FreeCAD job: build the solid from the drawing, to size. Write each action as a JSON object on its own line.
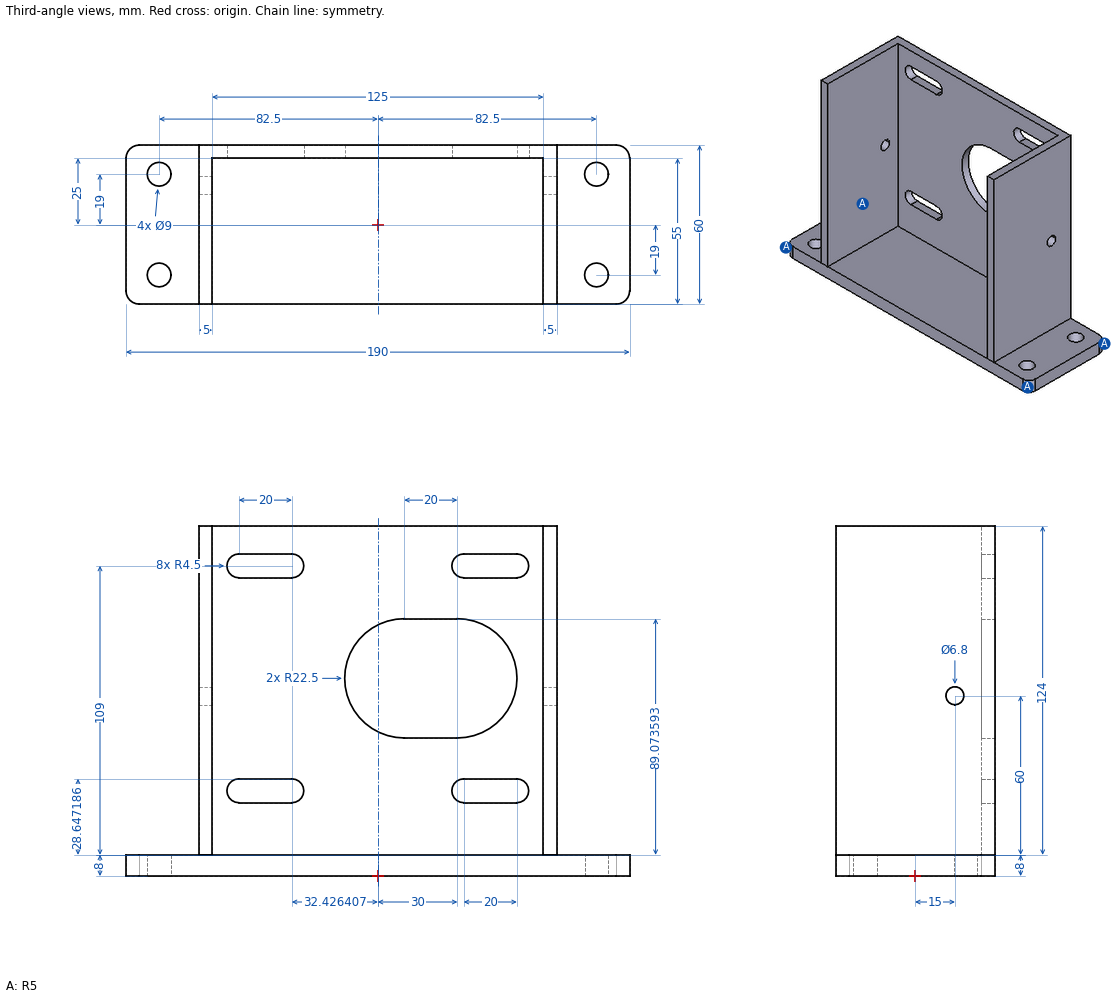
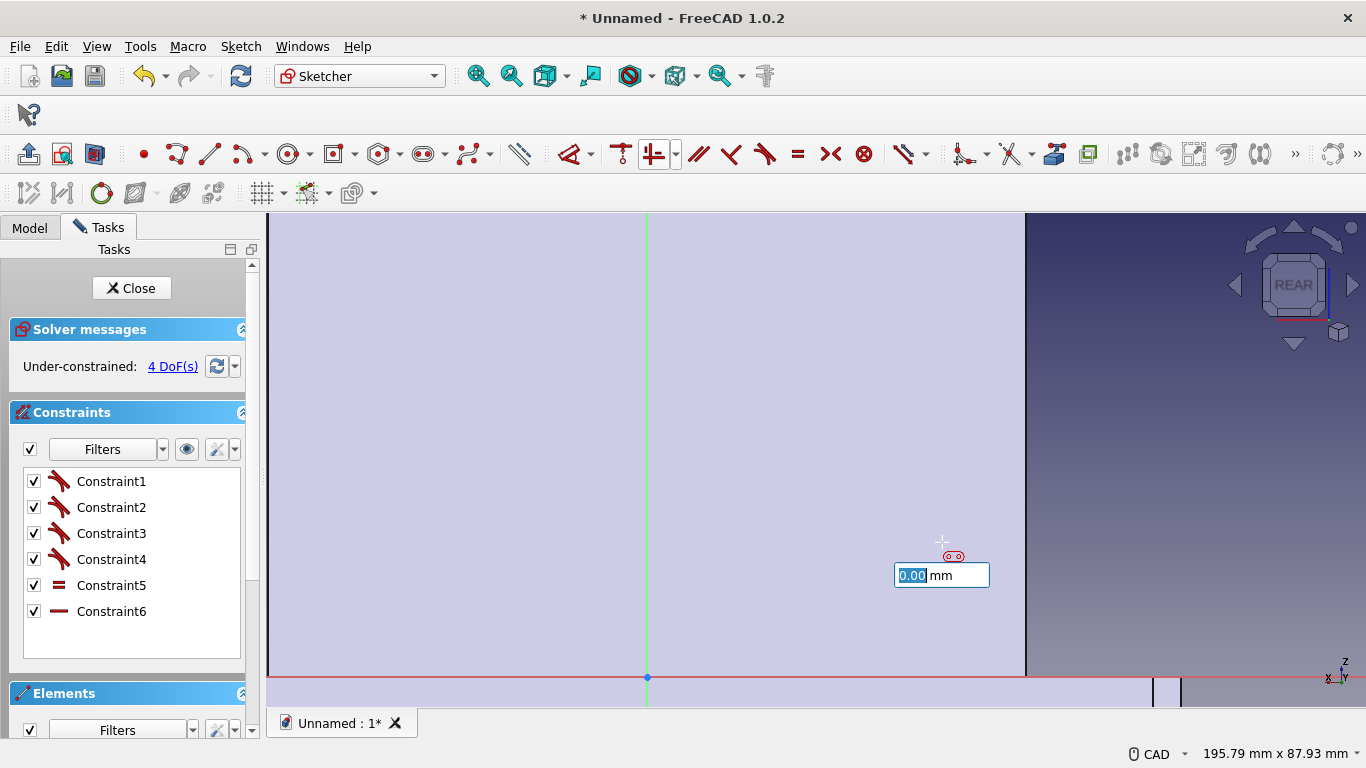
{"action": "left_click", "coordinate": [886, 516]}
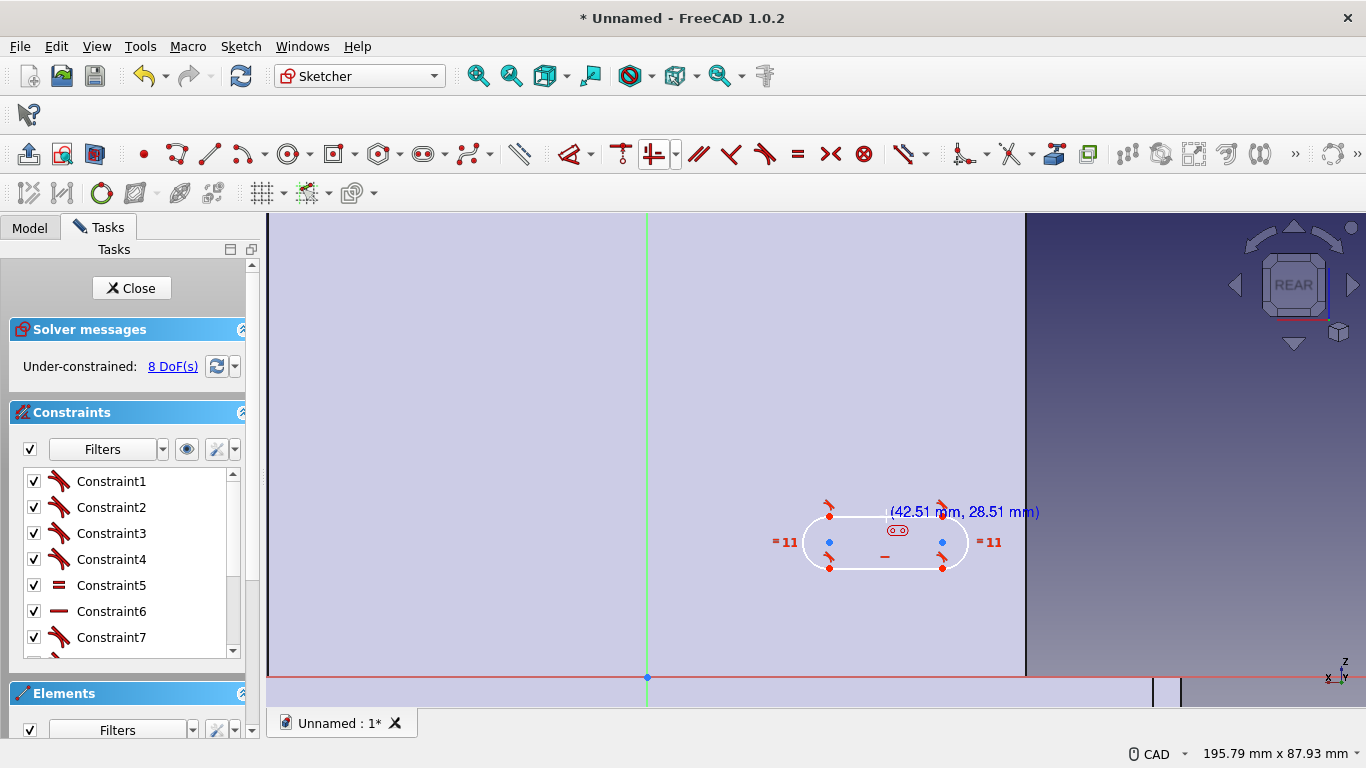
{"action": "left_click", "coordinate": [353, 542]}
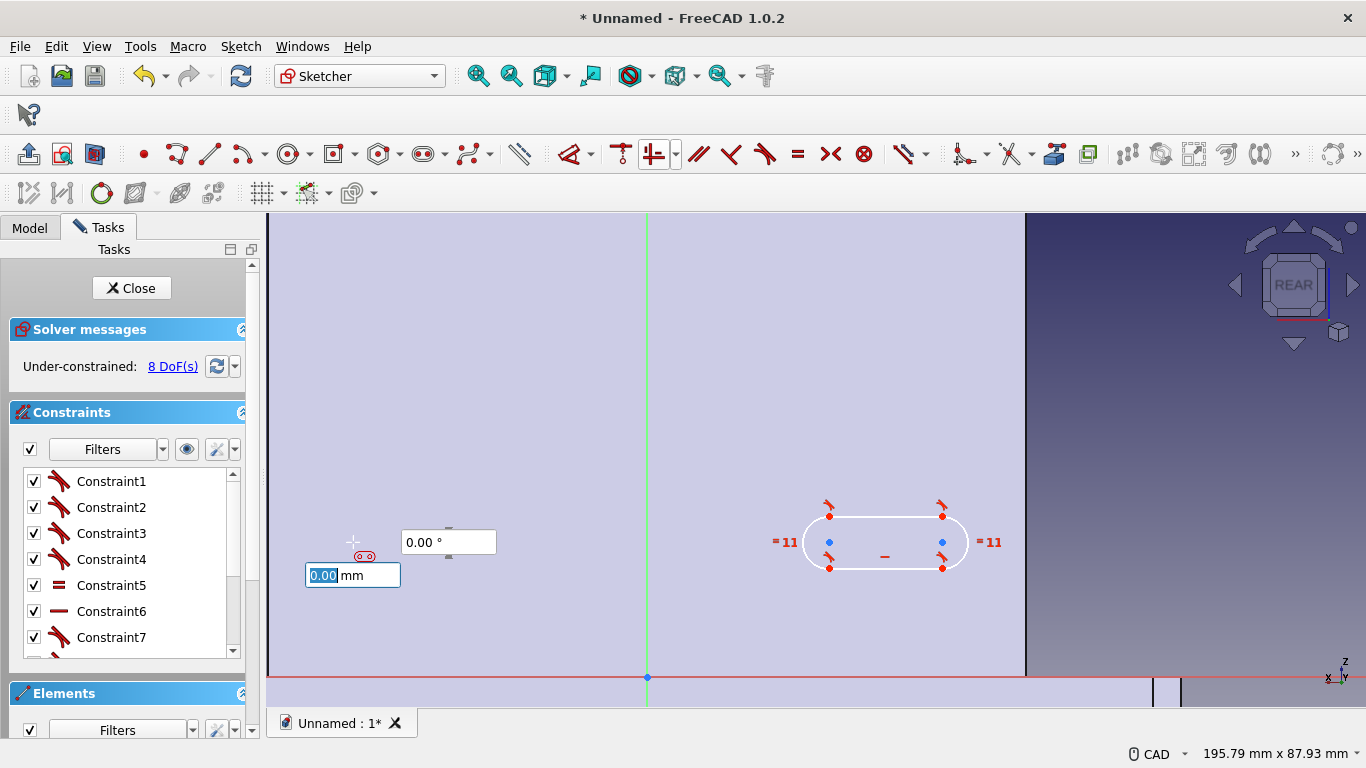
{"action": "left_click", "coordinate": [465, 542]}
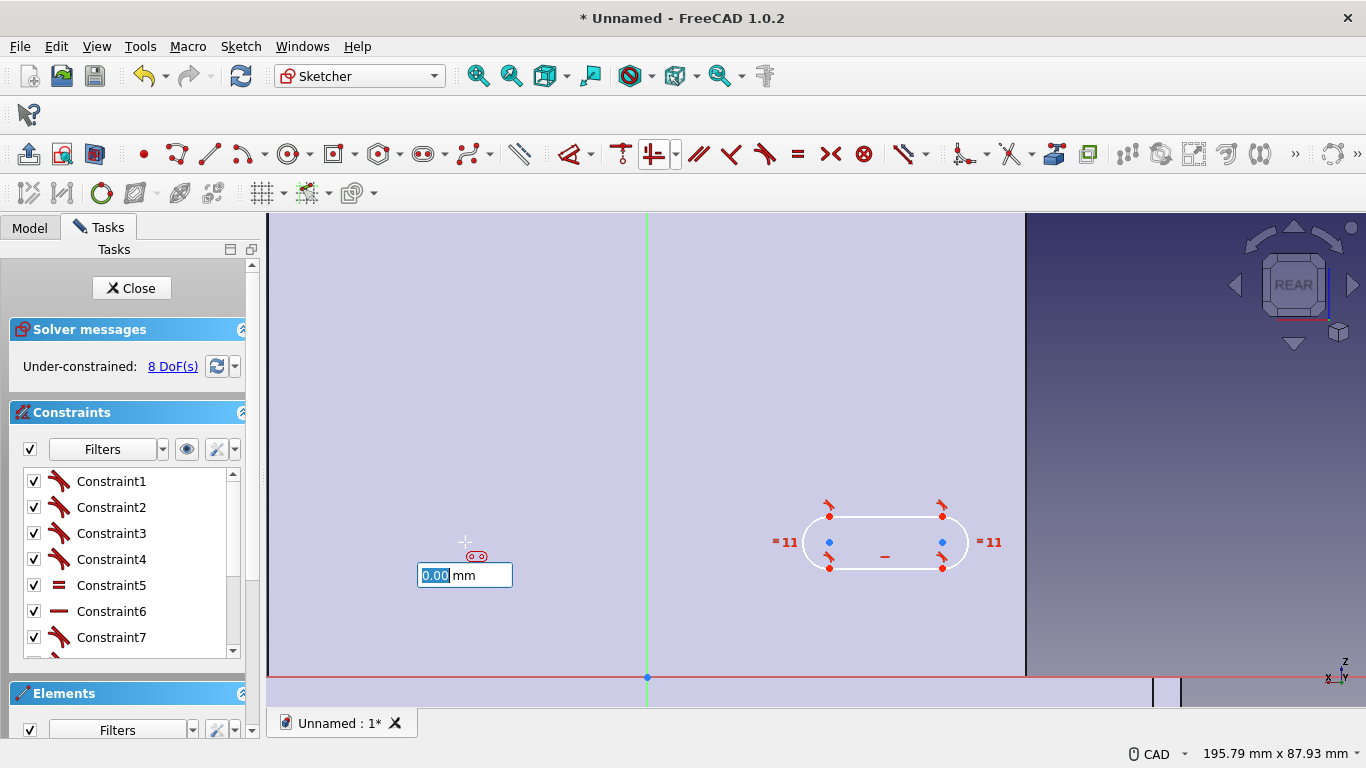
{"action": "left_click", "coordinate": [409, 567]}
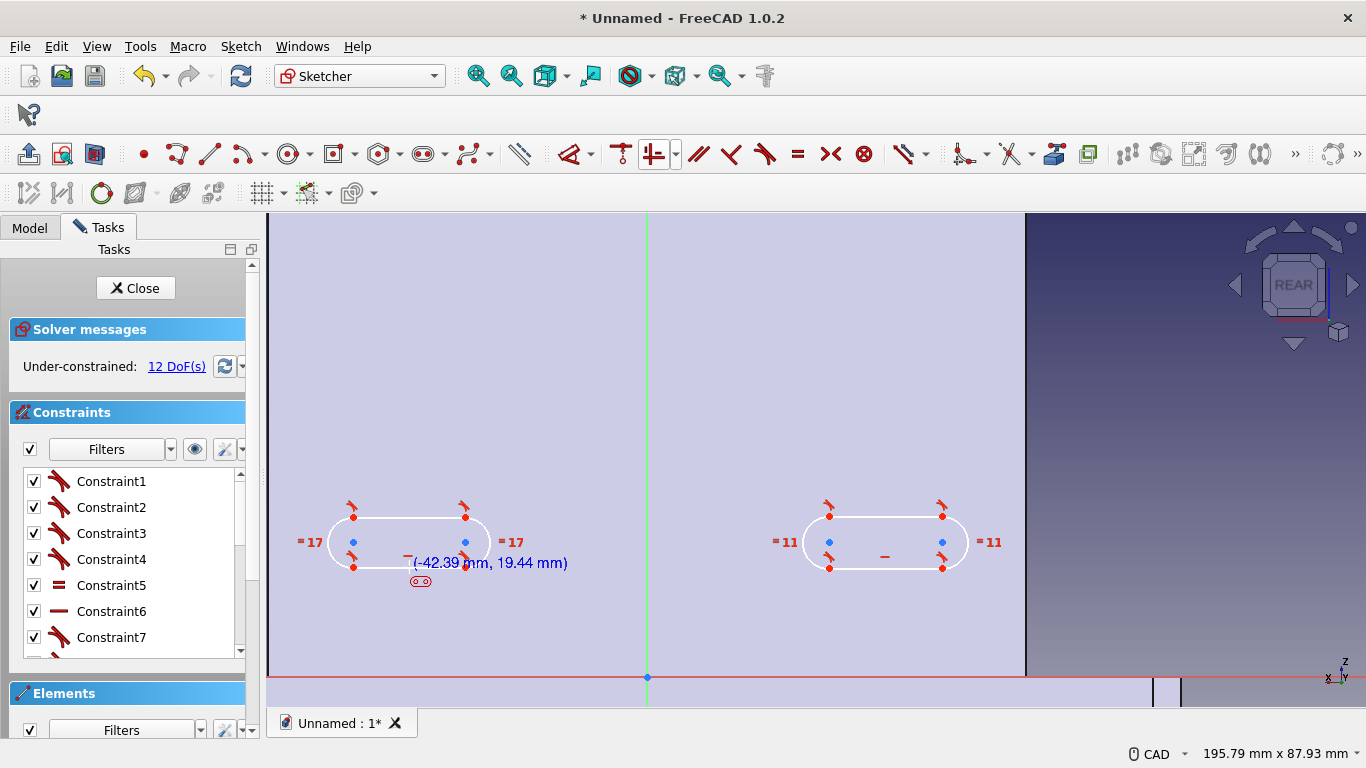
{"action": "scroll", "coordinate": [829, 543], "scroll_direction": "down", "scroll_amount": 4}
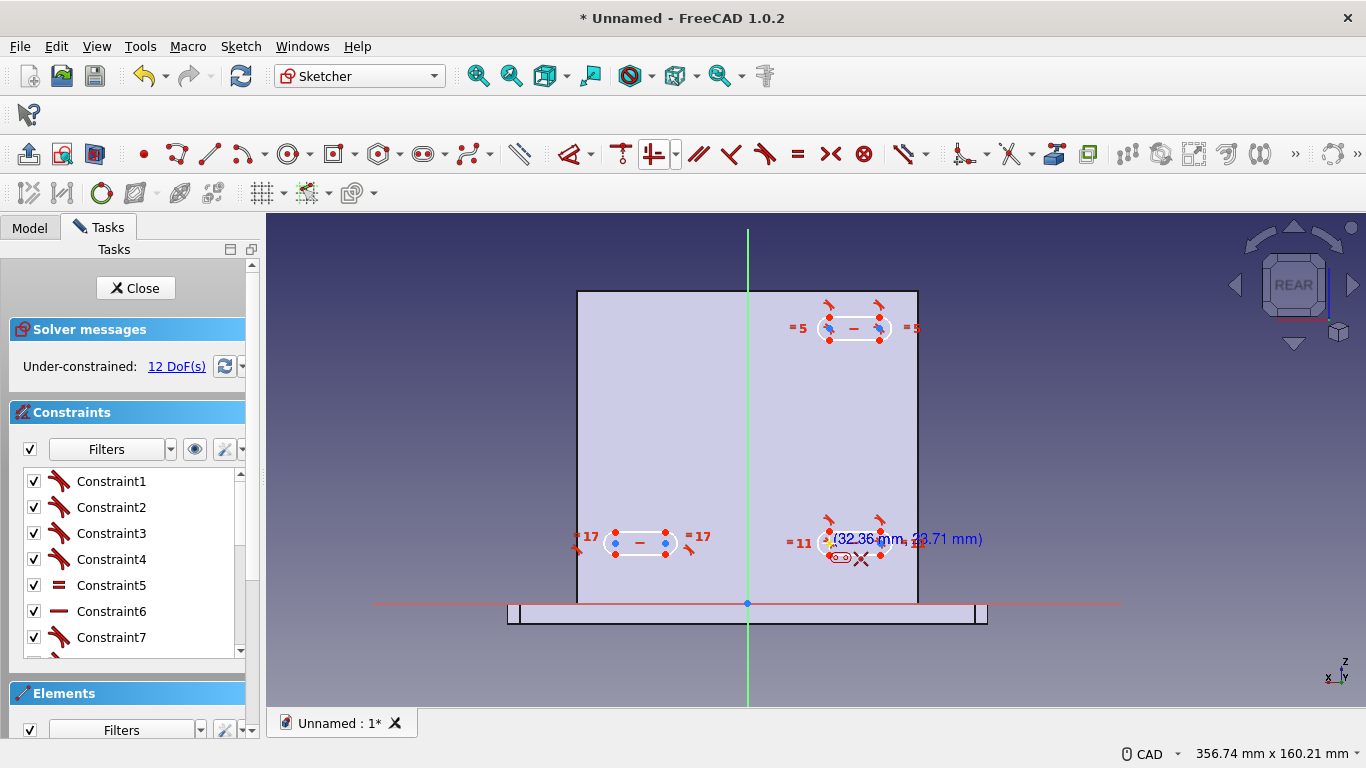
{"action": "scroll", "coordinate": [615, 328], "scroll_direction": "up", "scroll_amount": 4}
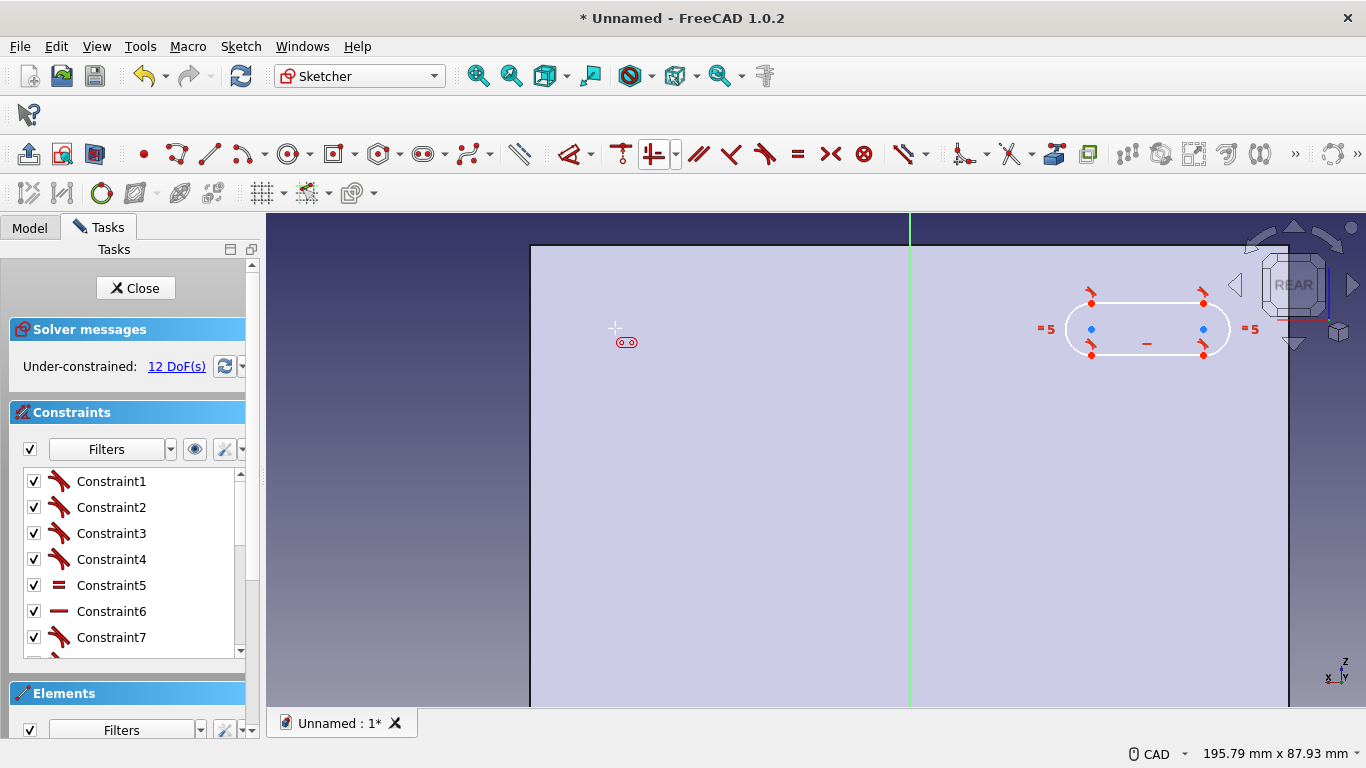
{"action": "left_click", "coordinate": [615, 329]}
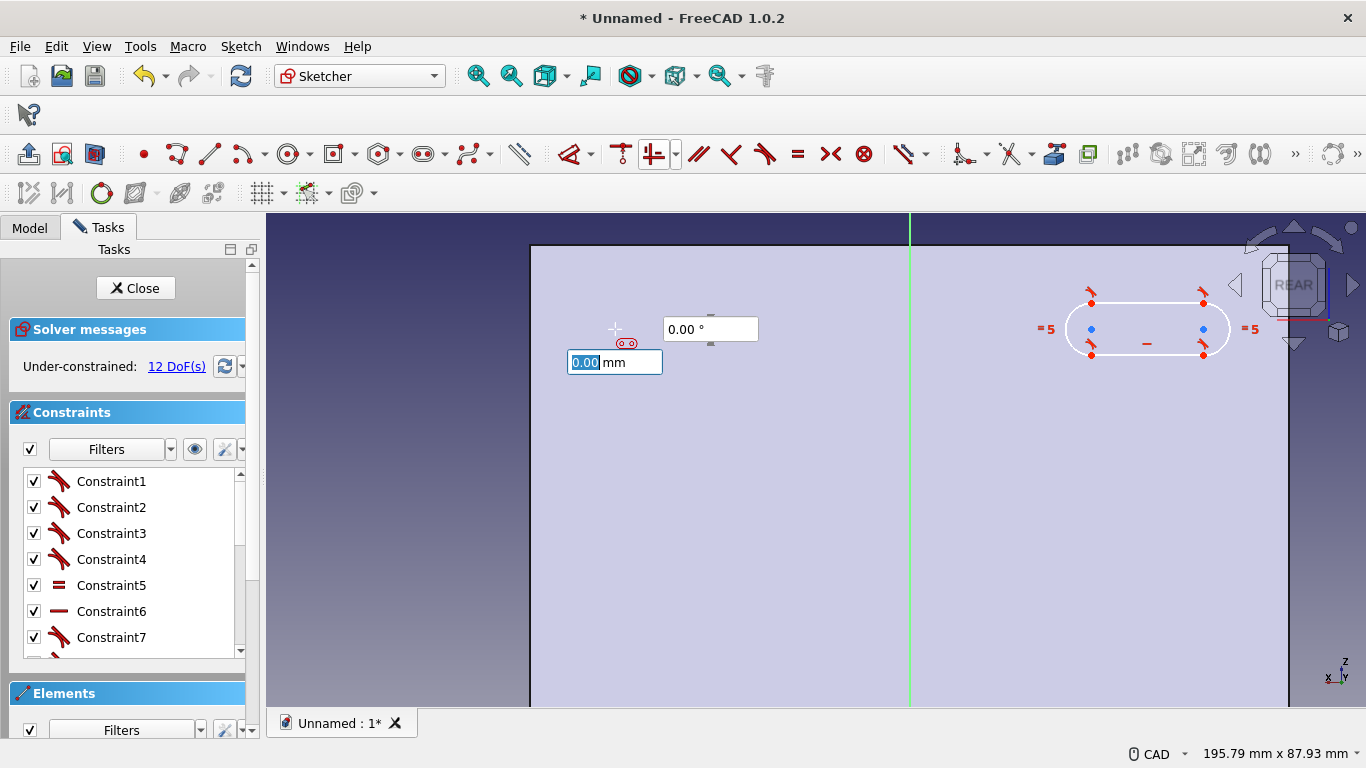
{"action": "left_click", "coordinate": [727, 329]}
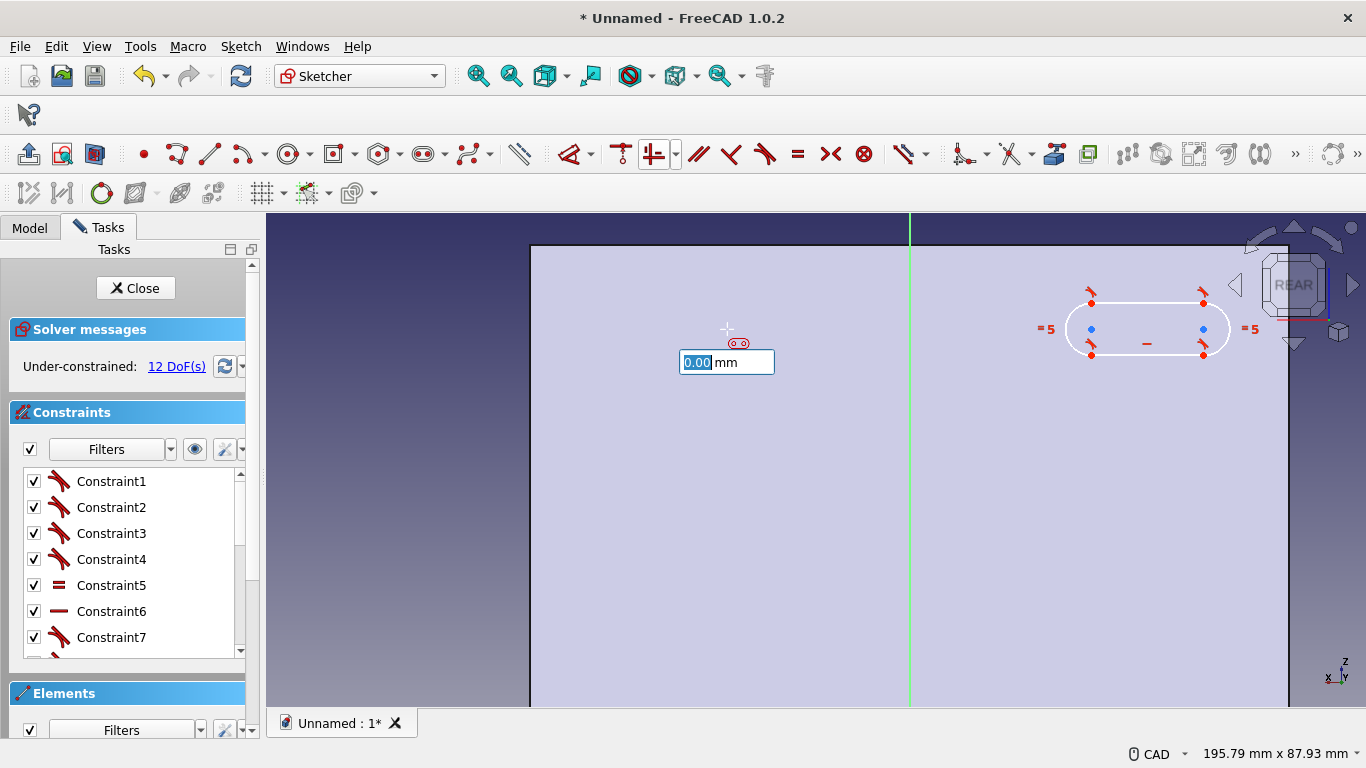
{"action": "left_click", "coordinate": [671, 354]}